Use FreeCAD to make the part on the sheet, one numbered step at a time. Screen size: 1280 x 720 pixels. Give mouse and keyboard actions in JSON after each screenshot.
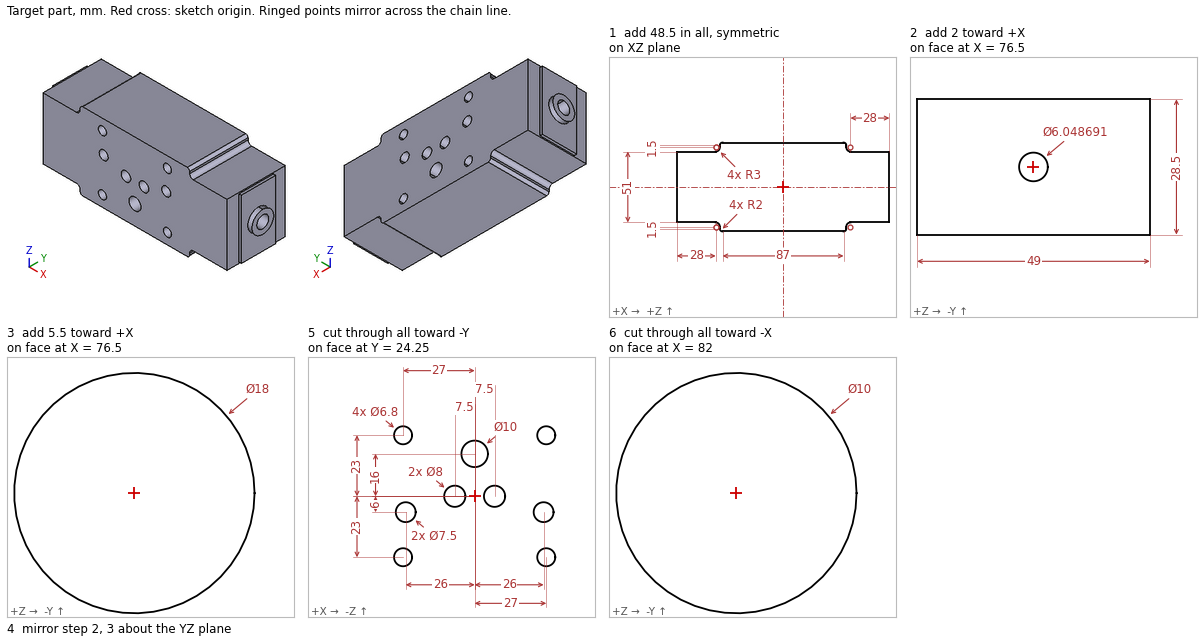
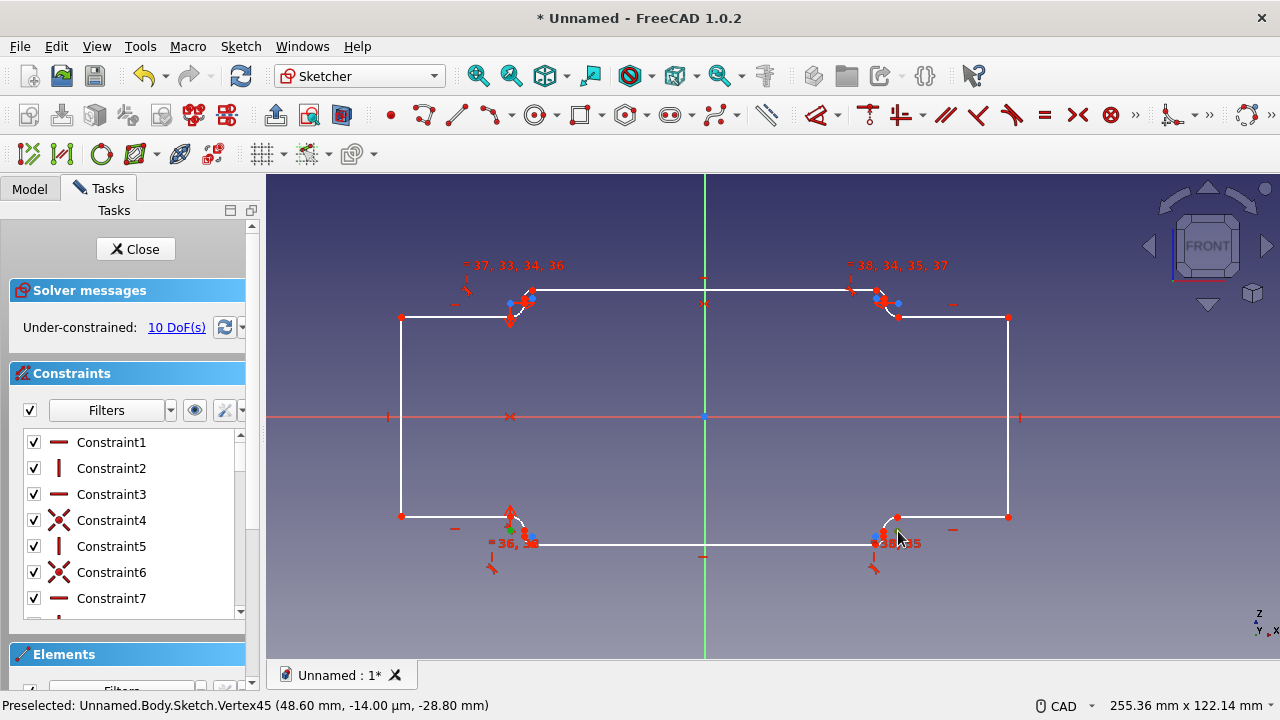
{"action": "left_click", "coordinate": [705, 600]}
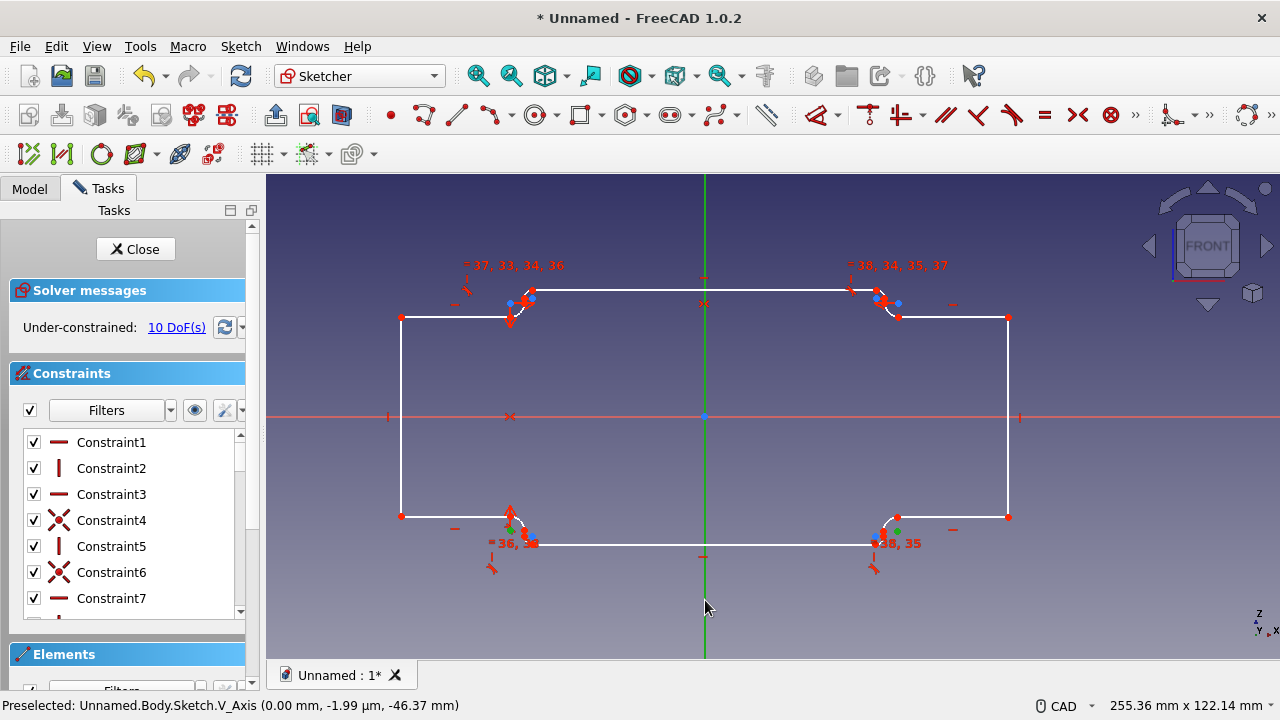
{"action": "key", "text": "s"}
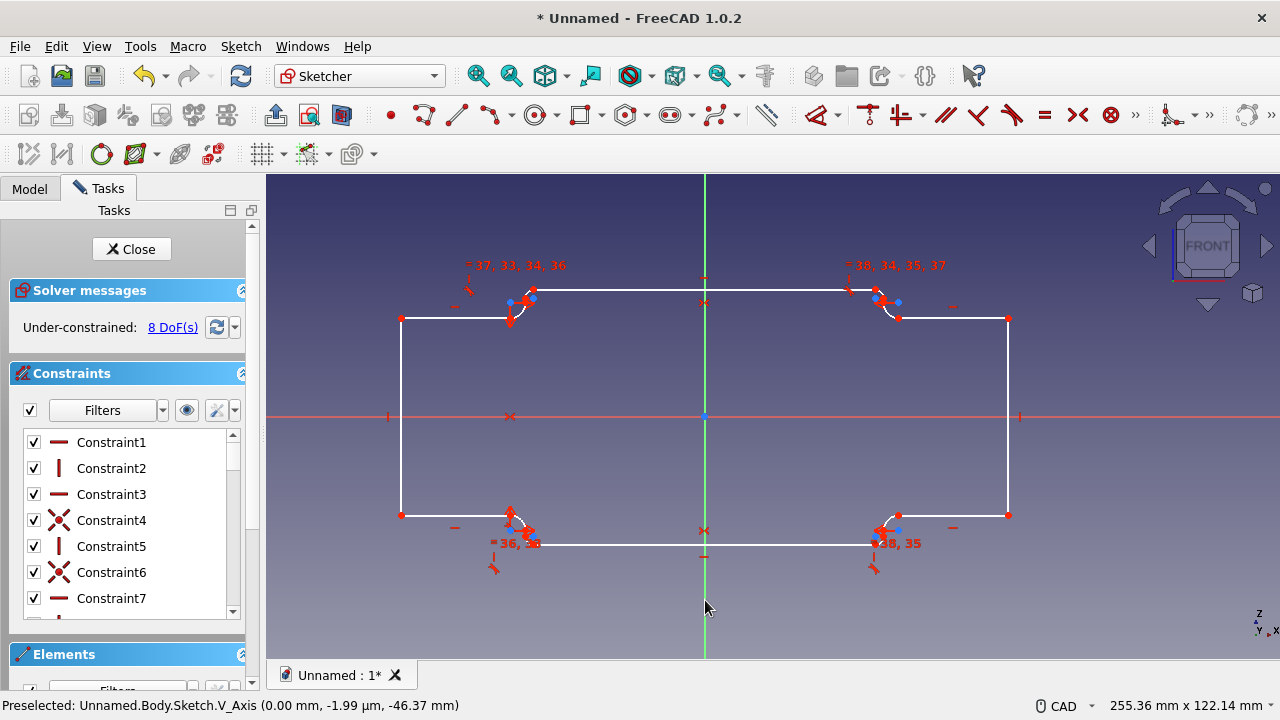
{"action": "scroll", "coordinate": [528, 542], "scroll_direction": "up", "scroll_amount": 9}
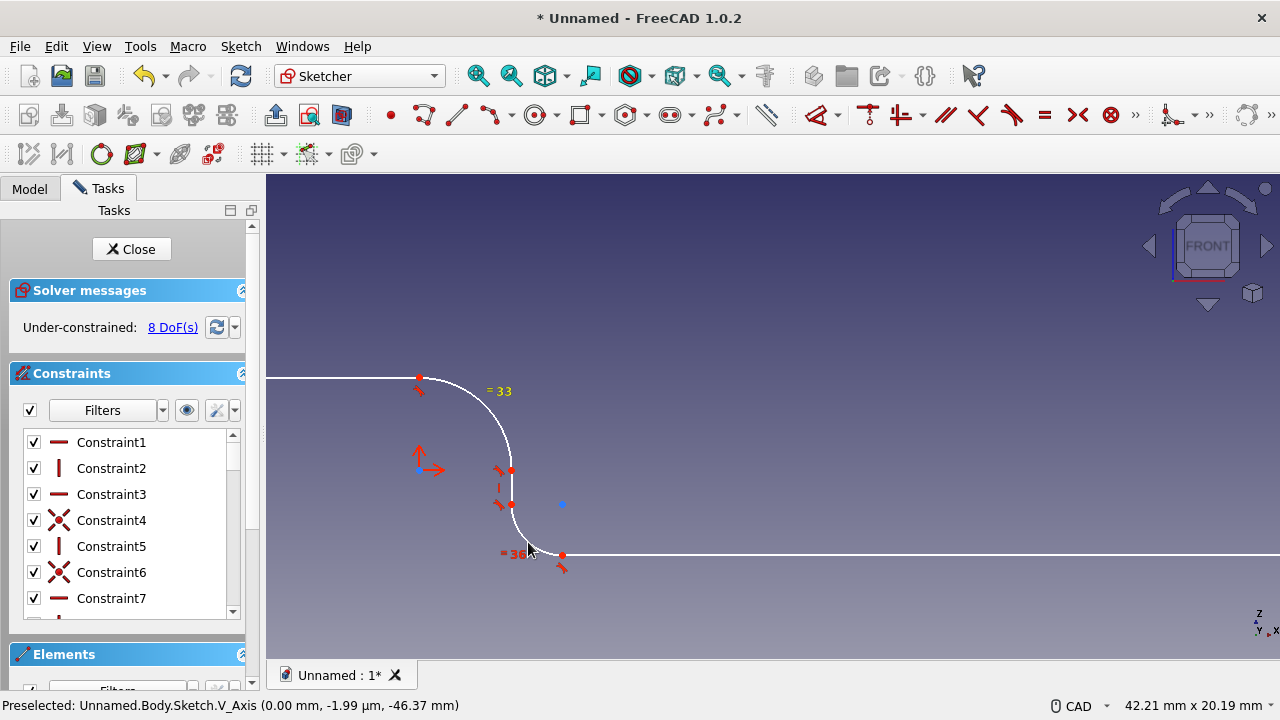
{"action": "left_click", "coordinate": [527, 540]}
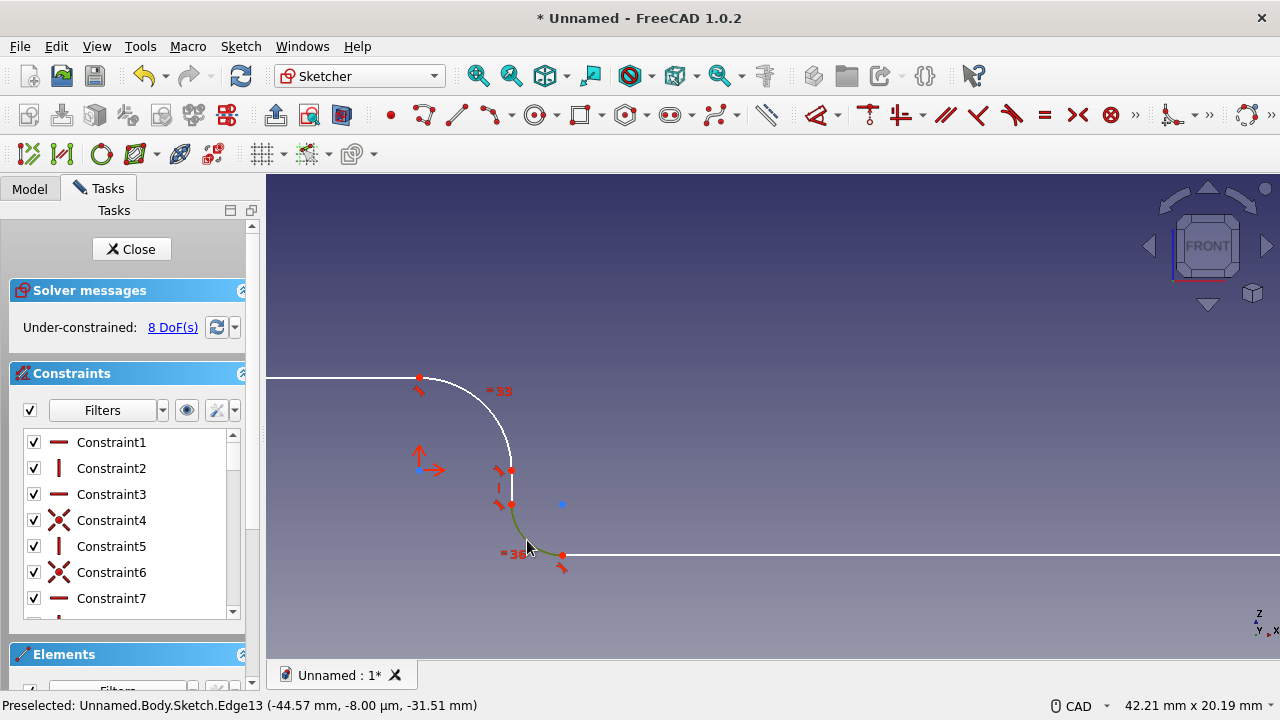
{"action": "key", "text": "k r"}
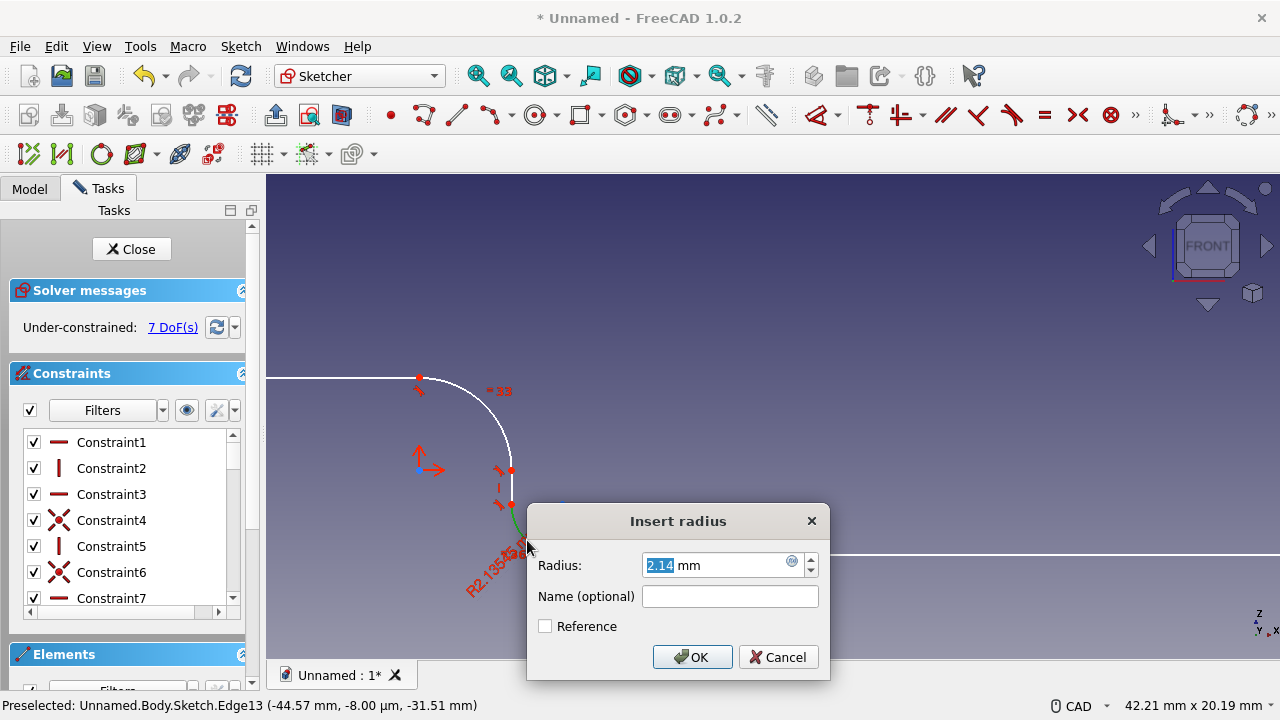
{"action": "type", "text": "2"}
{"action": "key", "text": "Return"}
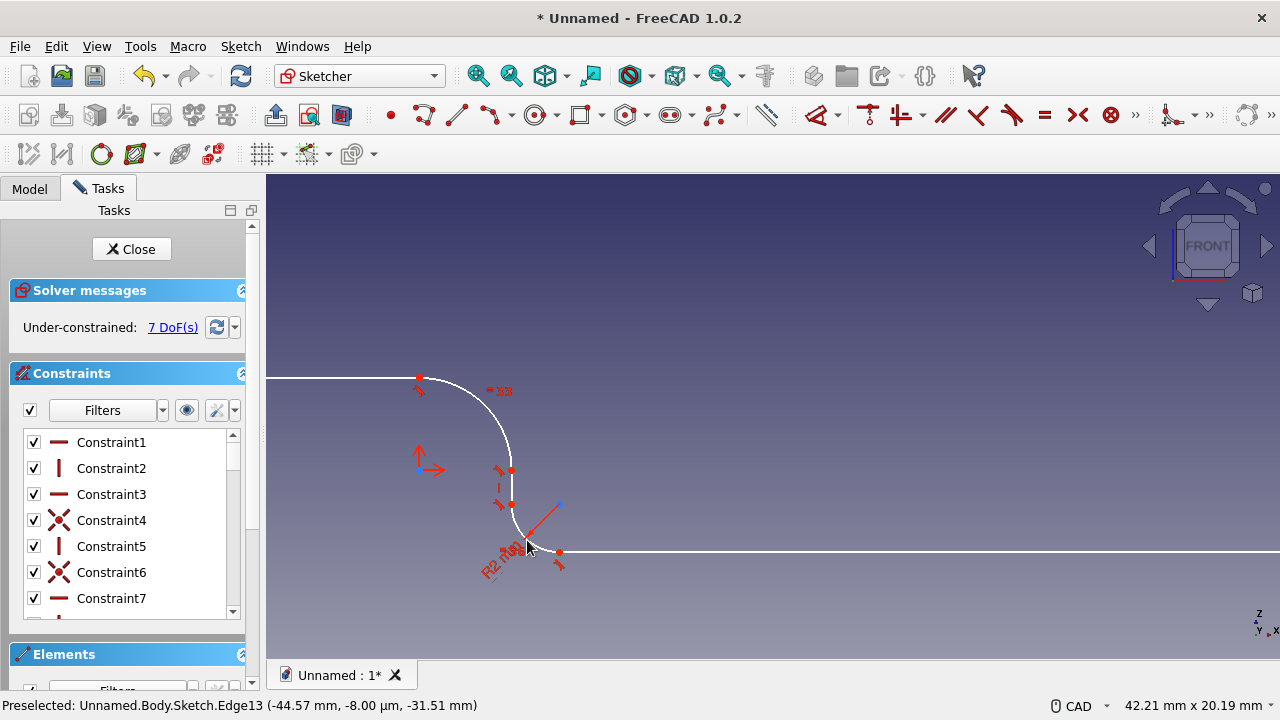
{"action": "left_click", "coordinate": [502, 428]}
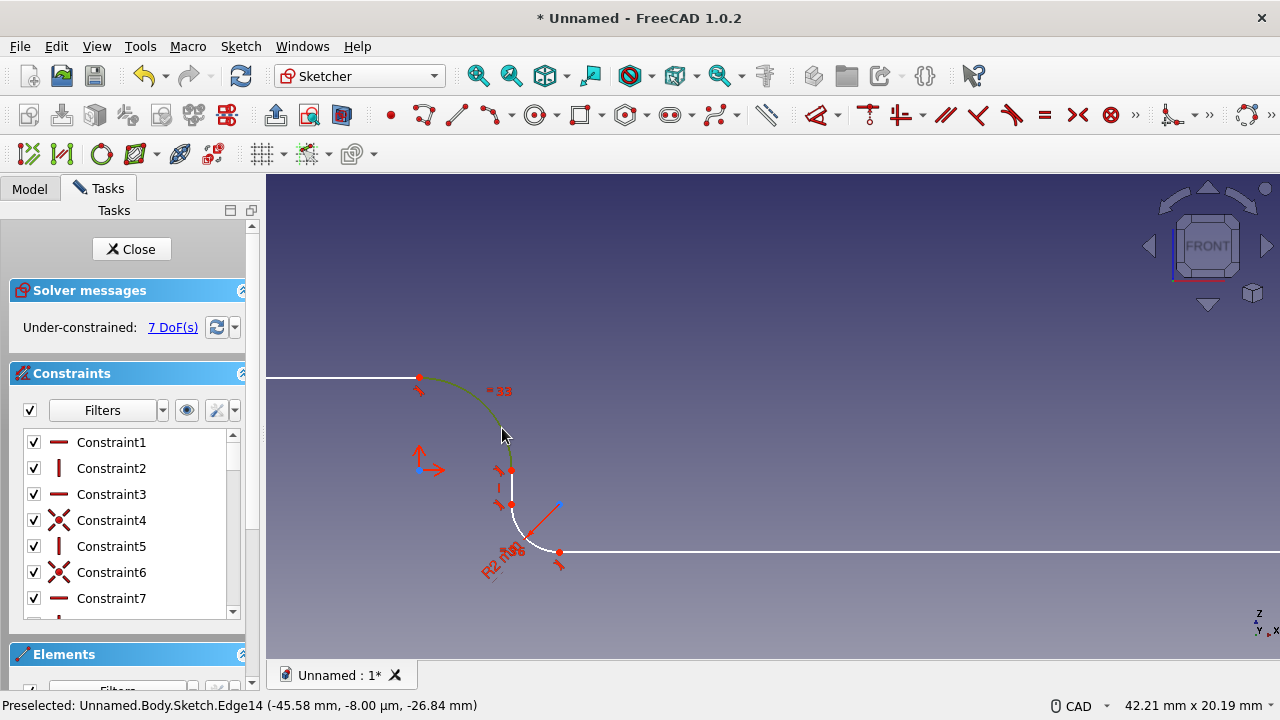
{"action": "key", "text": "k r"}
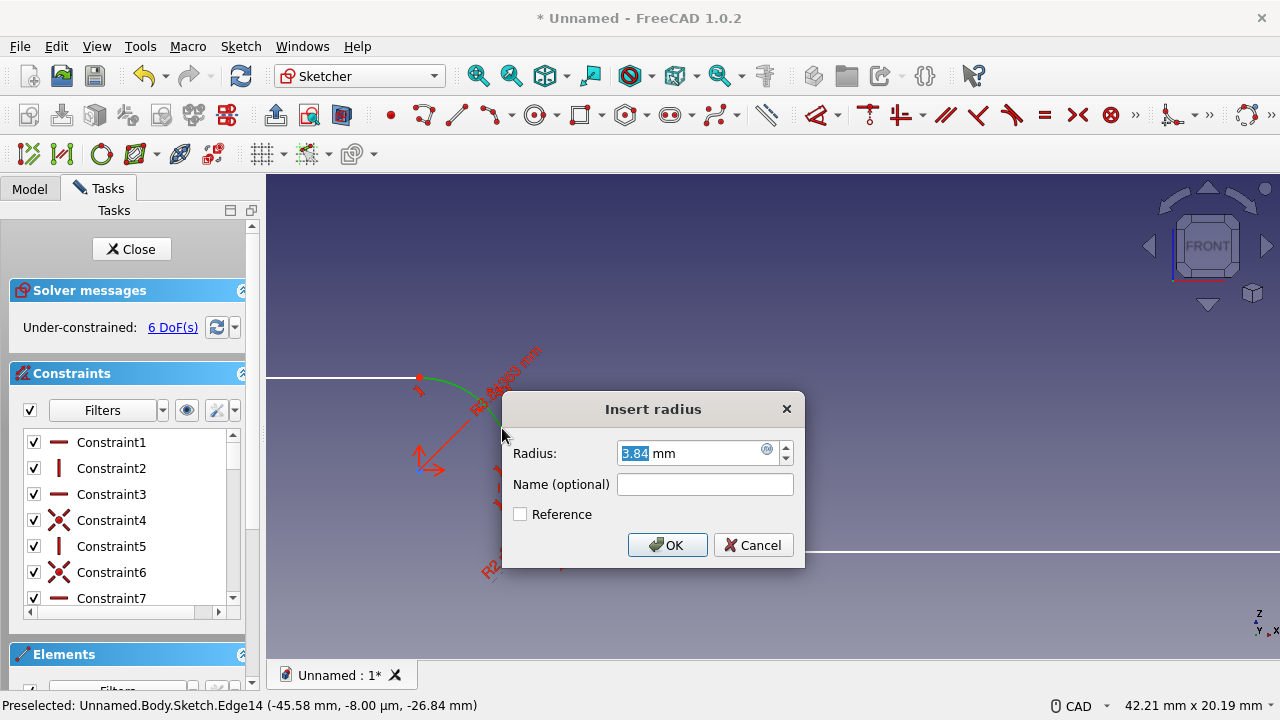
{"action": "type", "text": "3"}
{"action": "key", "text": "Return"}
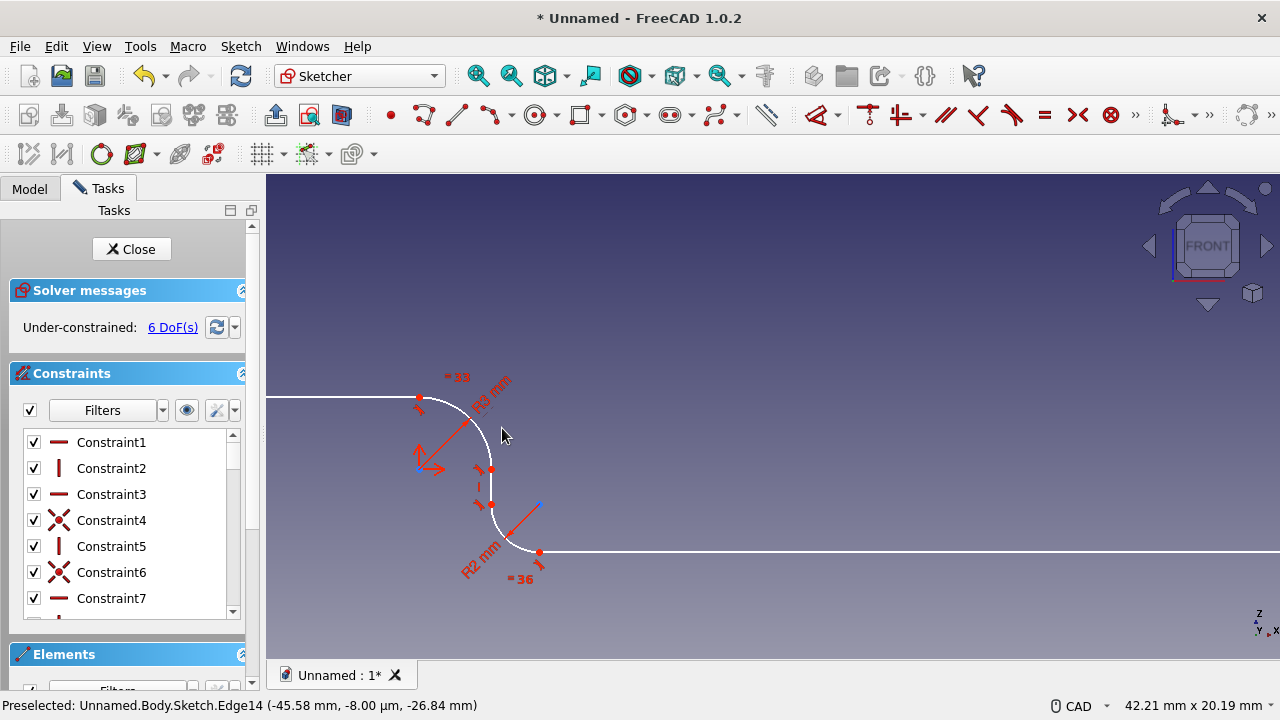
{"action": "scroll", "coordinate": [528, 542], "scroll_direction": "down", "scroll_amount": 9}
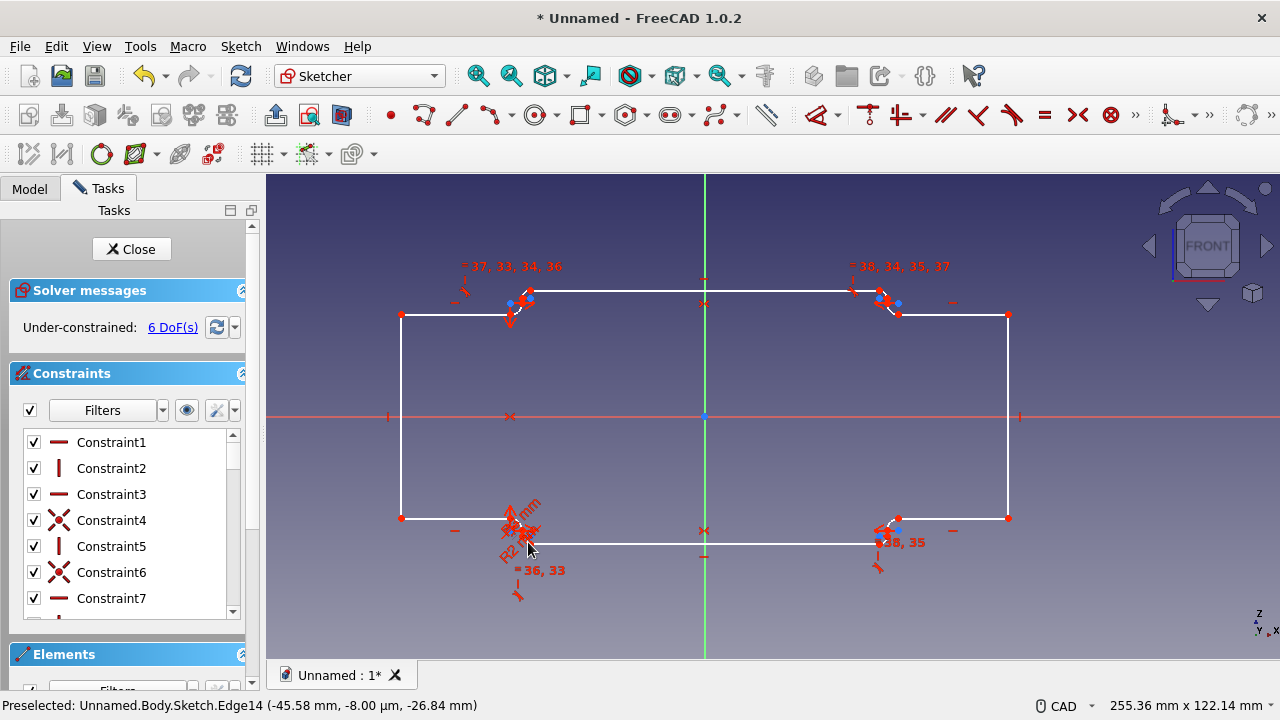
{"action": "left_click", "coordinate": [600, 544]}